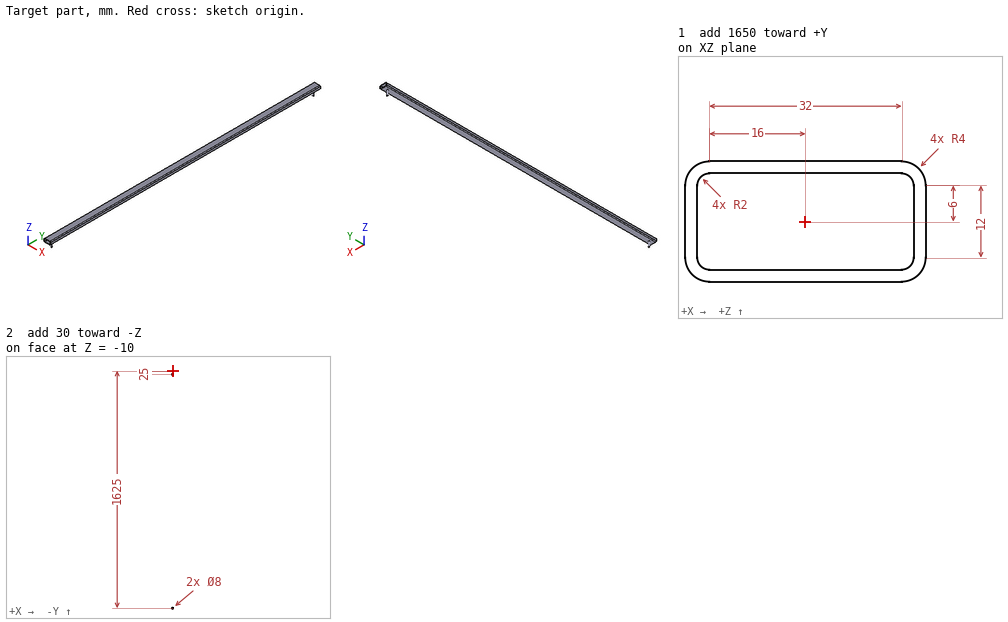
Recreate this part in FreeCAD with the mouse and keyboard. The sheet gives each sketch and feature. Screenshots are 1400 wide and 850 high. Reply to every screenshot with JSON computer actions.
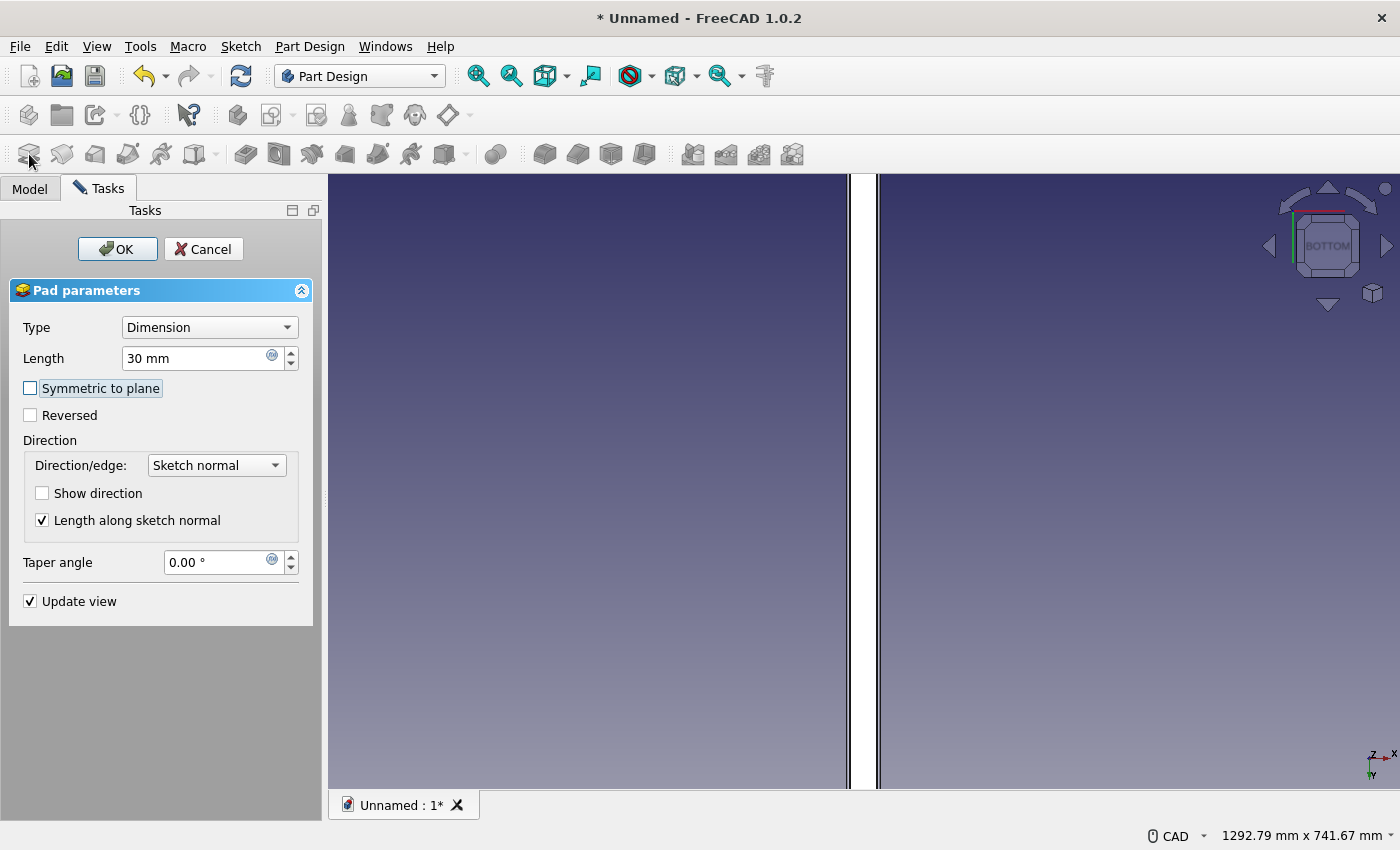
{"action": "left_click", "coordinate": [118, 249]}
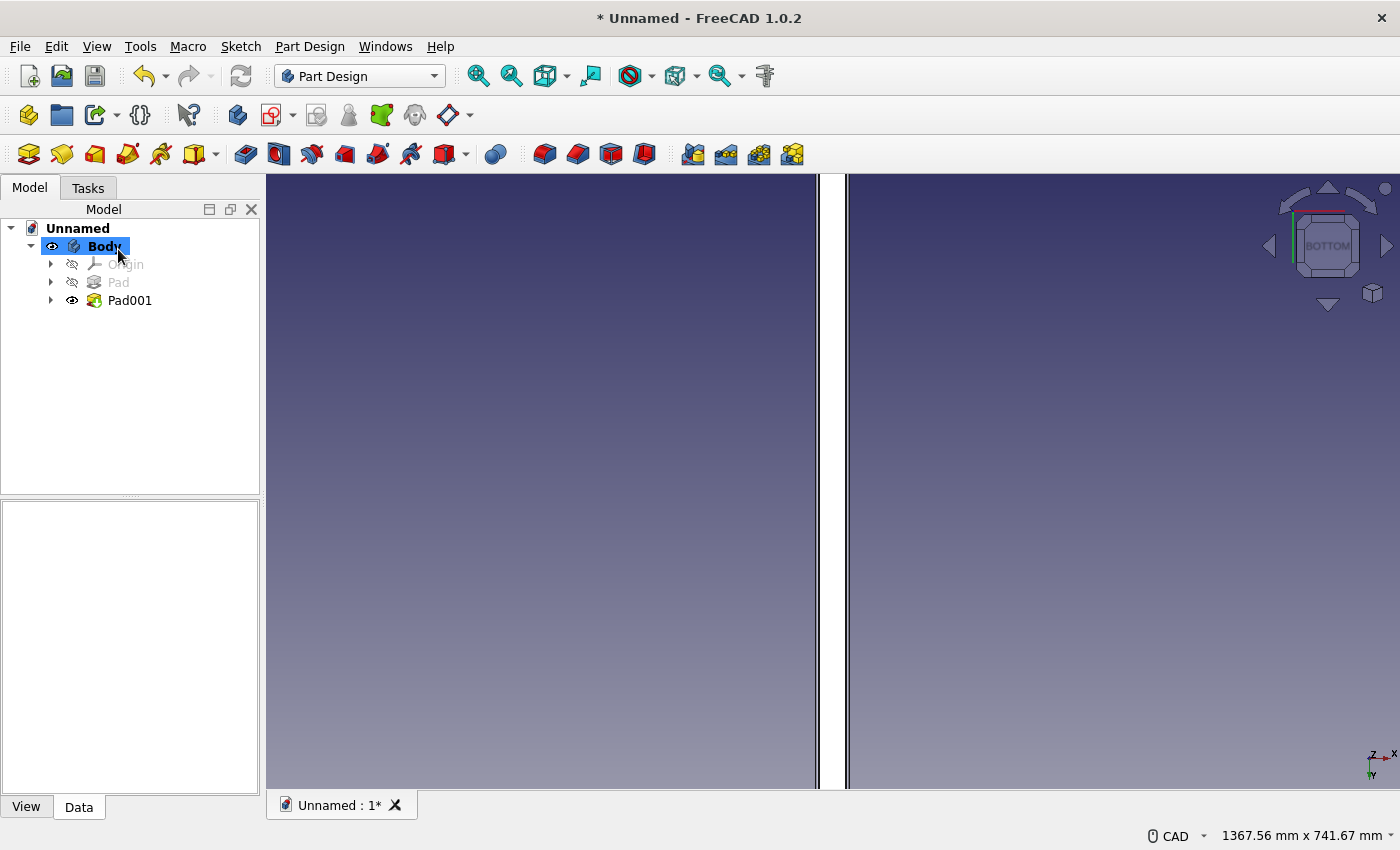
{"action": "key", "text": "0"}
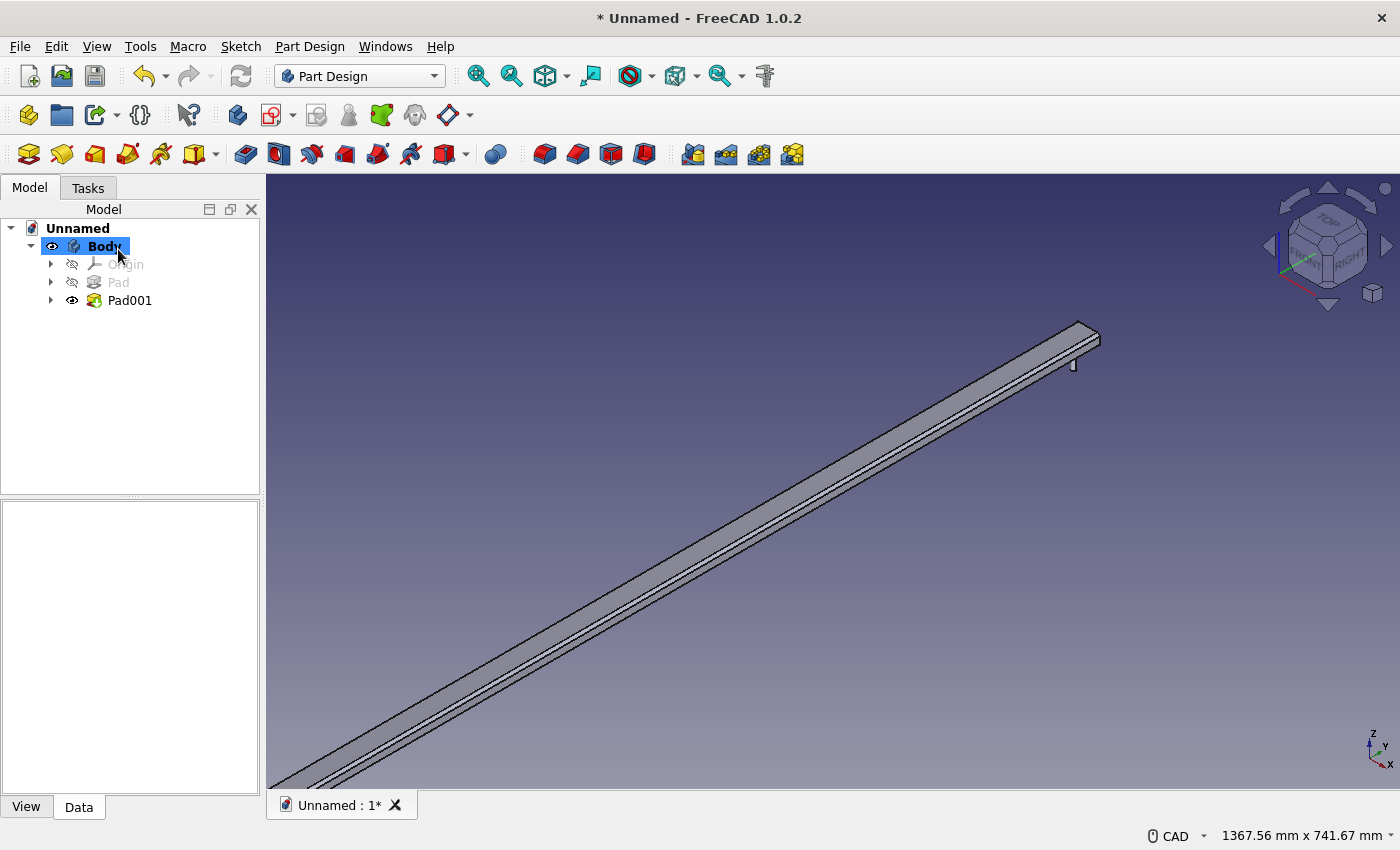
{"action": "left_click", "coordinate": [479, 76]}